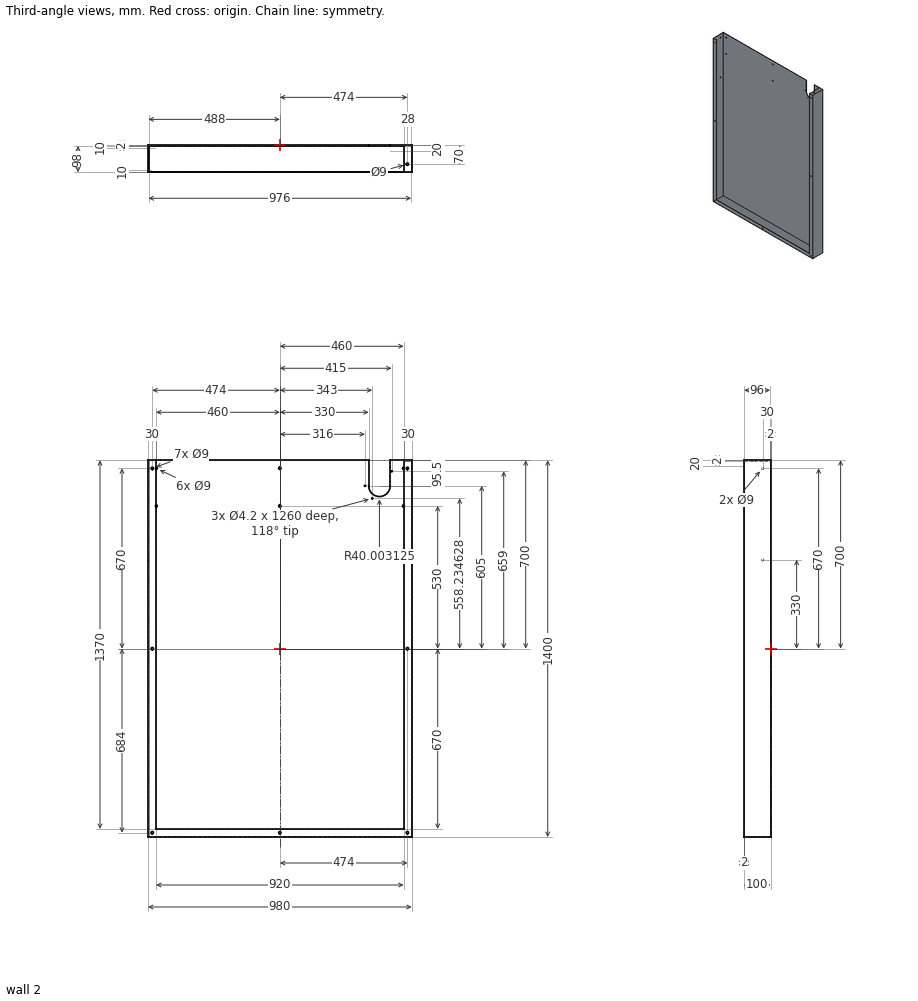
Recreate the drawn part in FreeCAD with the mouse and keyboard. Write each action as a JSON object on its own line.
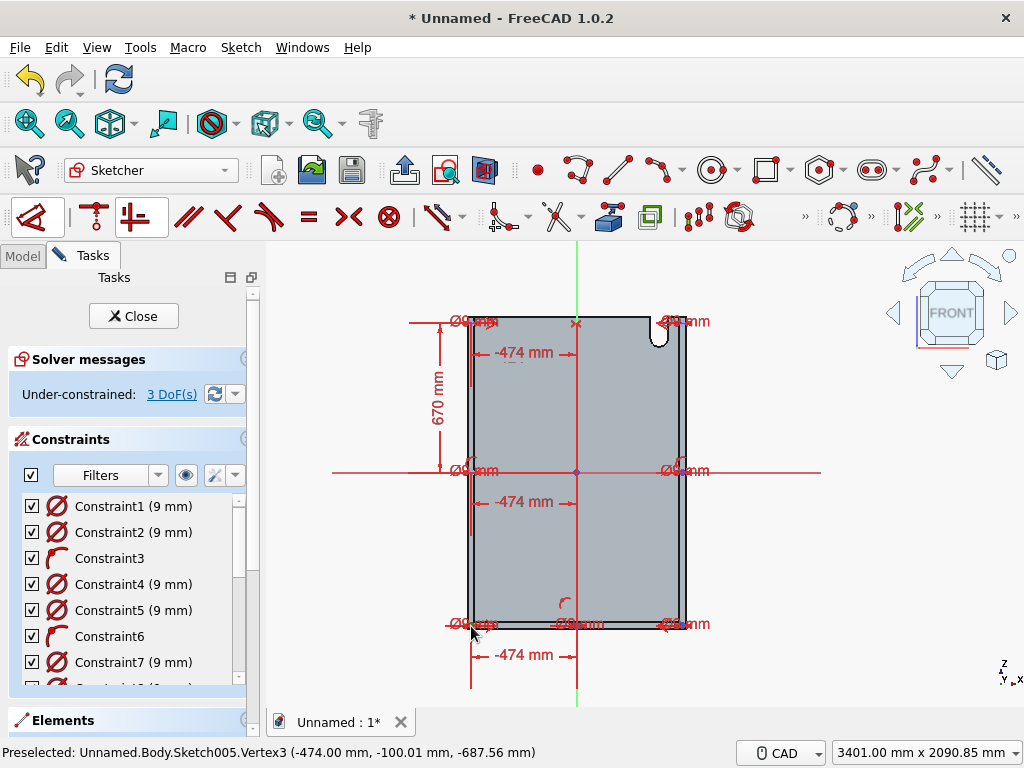
{"action": "key", "text": "i"}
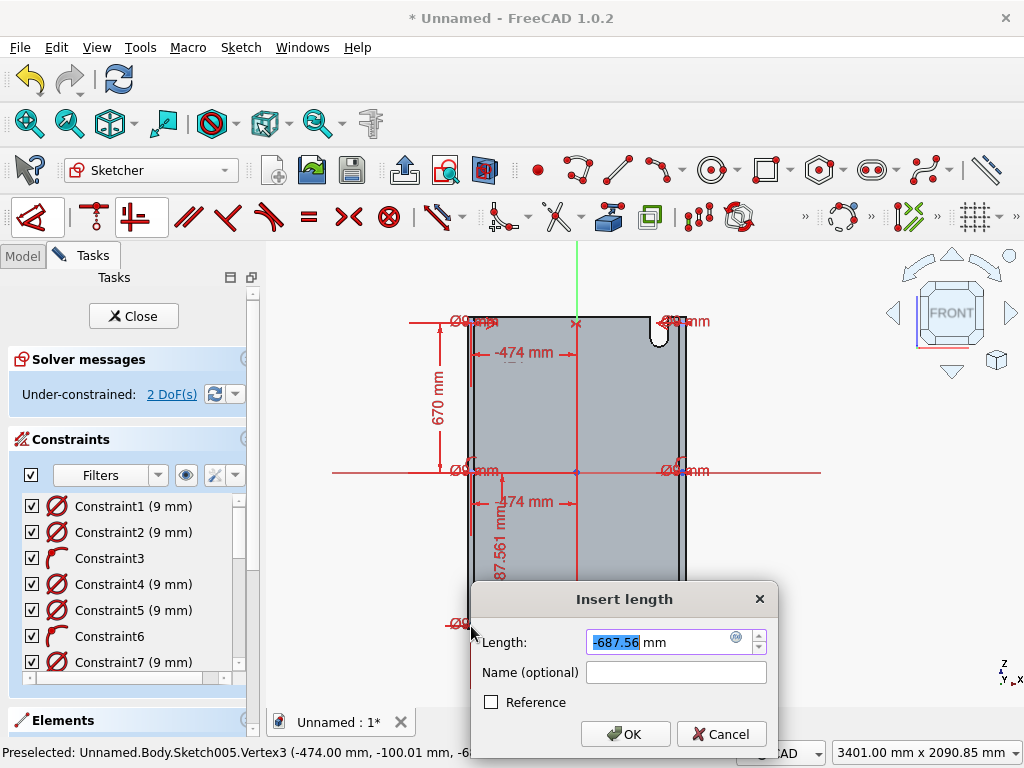
{"action": "type", "text": "-684"}
{"action": "key", "text": "Return"}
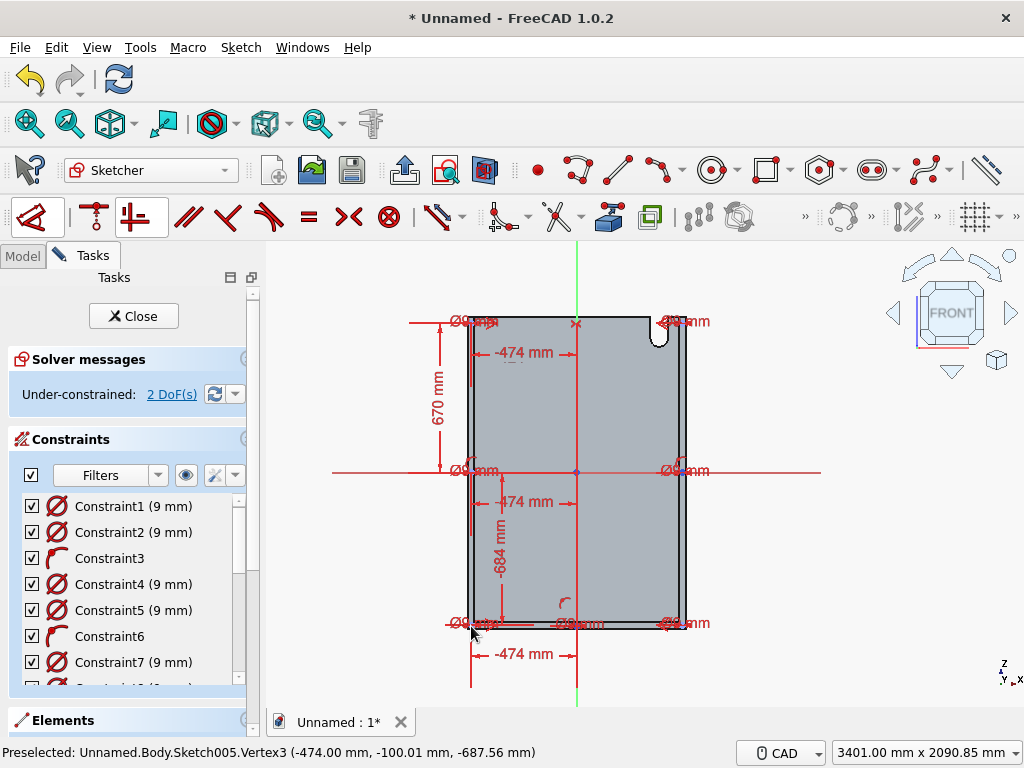
{"action": "left_click", "coordinate": [577, 626]}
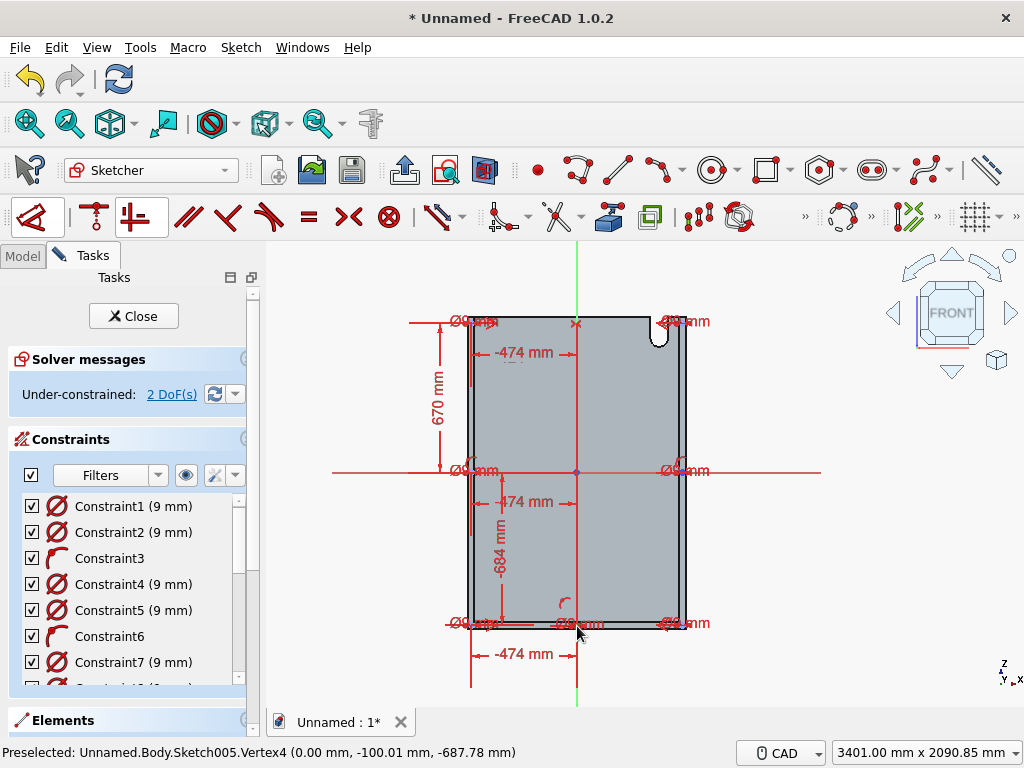
{"action": "key", "text": "i"}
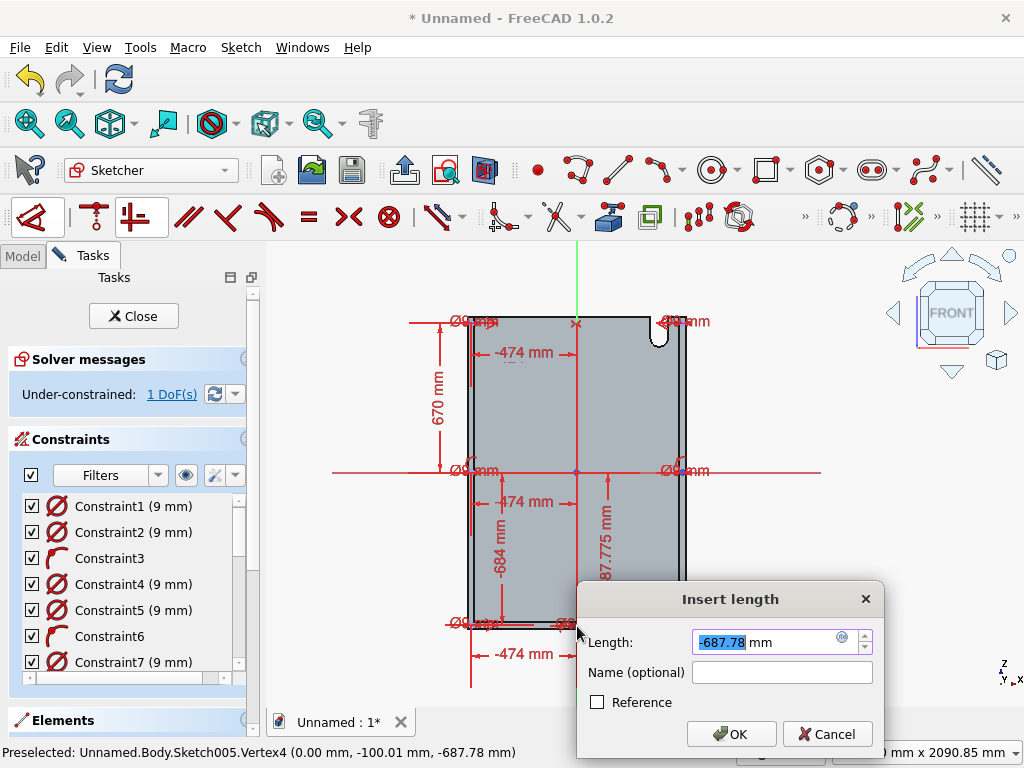
{"action": "type", "text": "-684"}
{"action": "key", "text": "Return"}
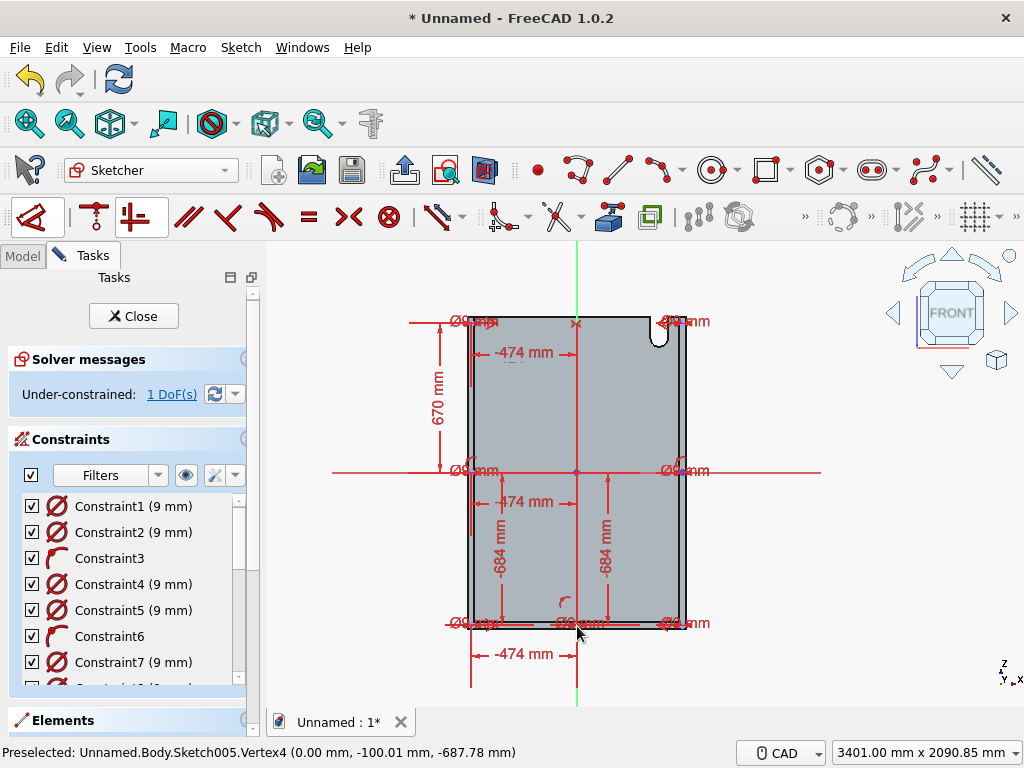
{"action": "left_click", "coordinate": [682, 473]}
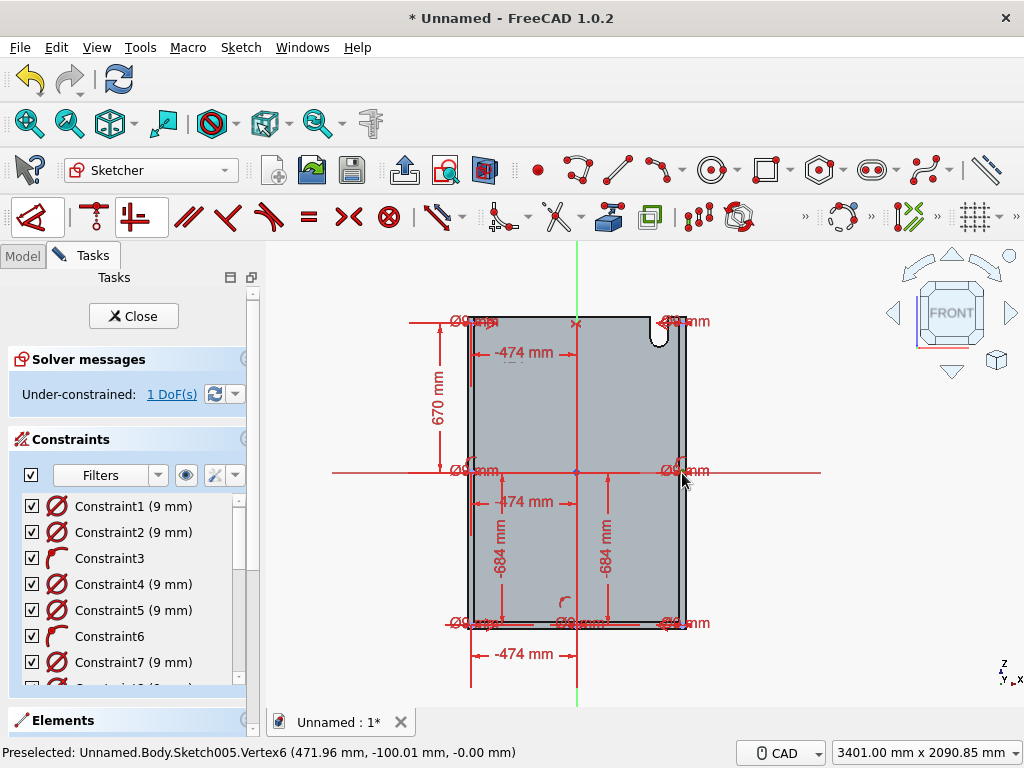
{"action": "left_click", "coordinate": [58, 218]}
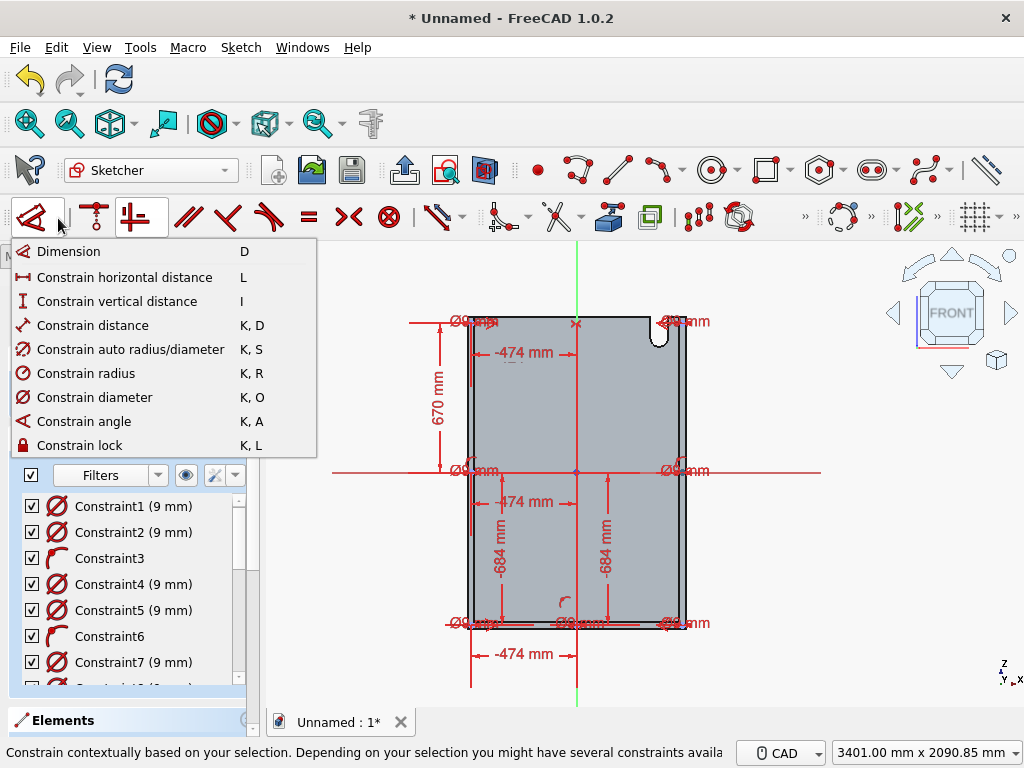
{"action": "left_click", "coordinate": [164, 277]}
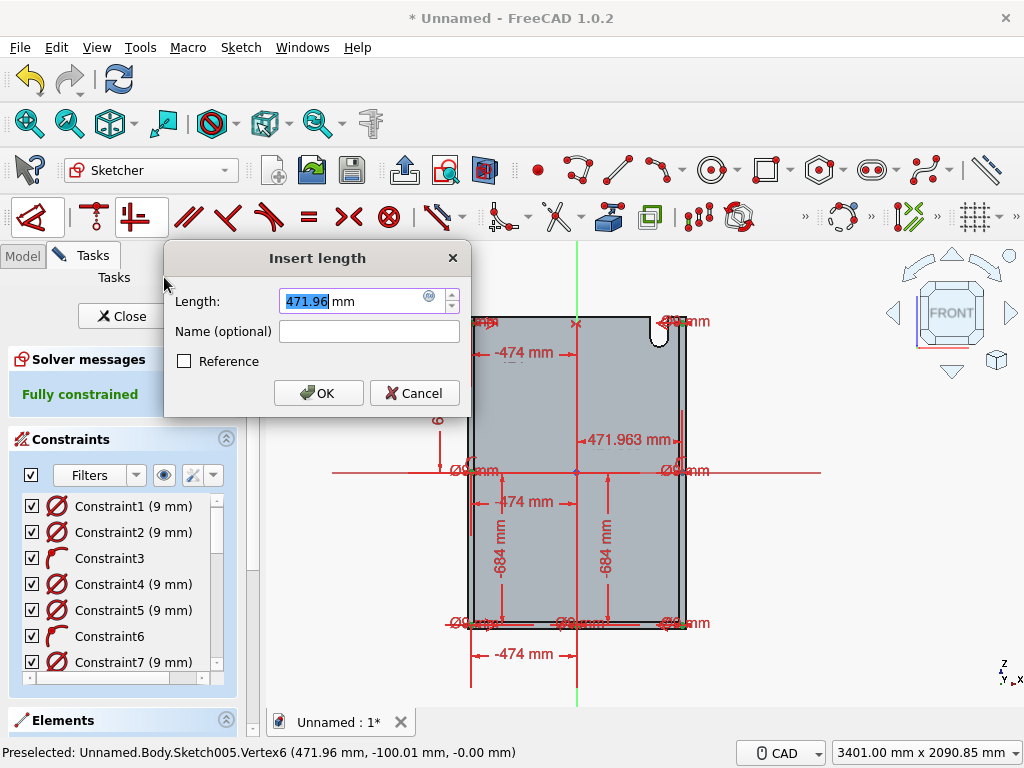
{"action": "type", "text": "474"}
{"action": "key", "text": "Return"}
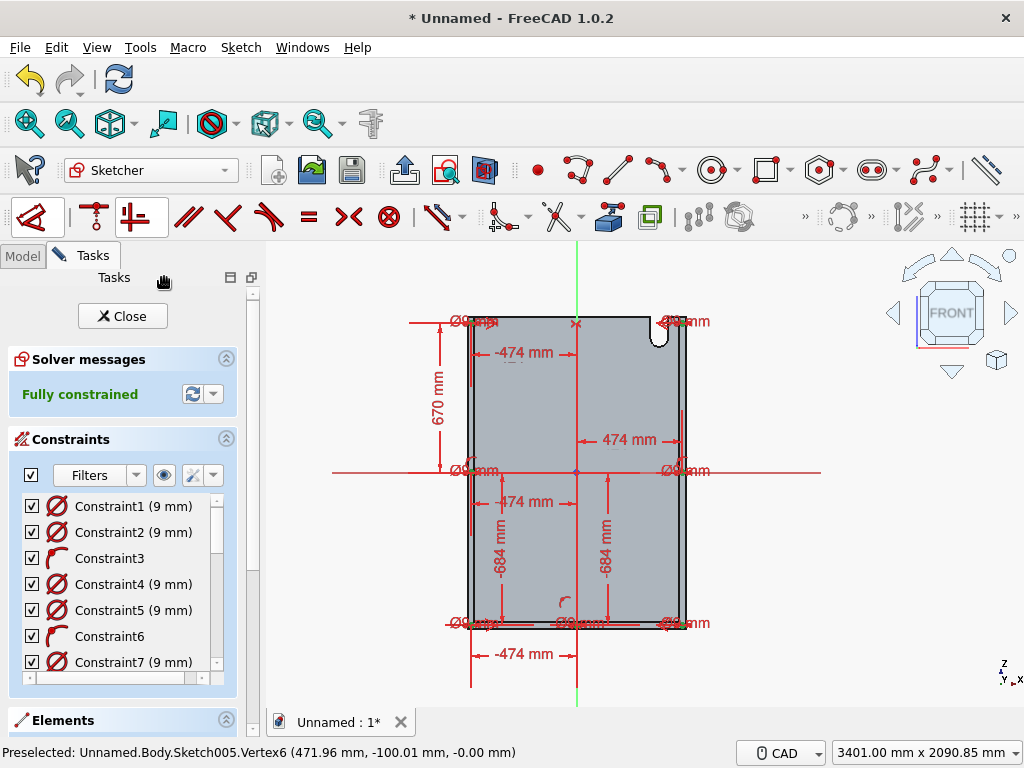
{"action": "left_click", "coordinate": [123, 316]}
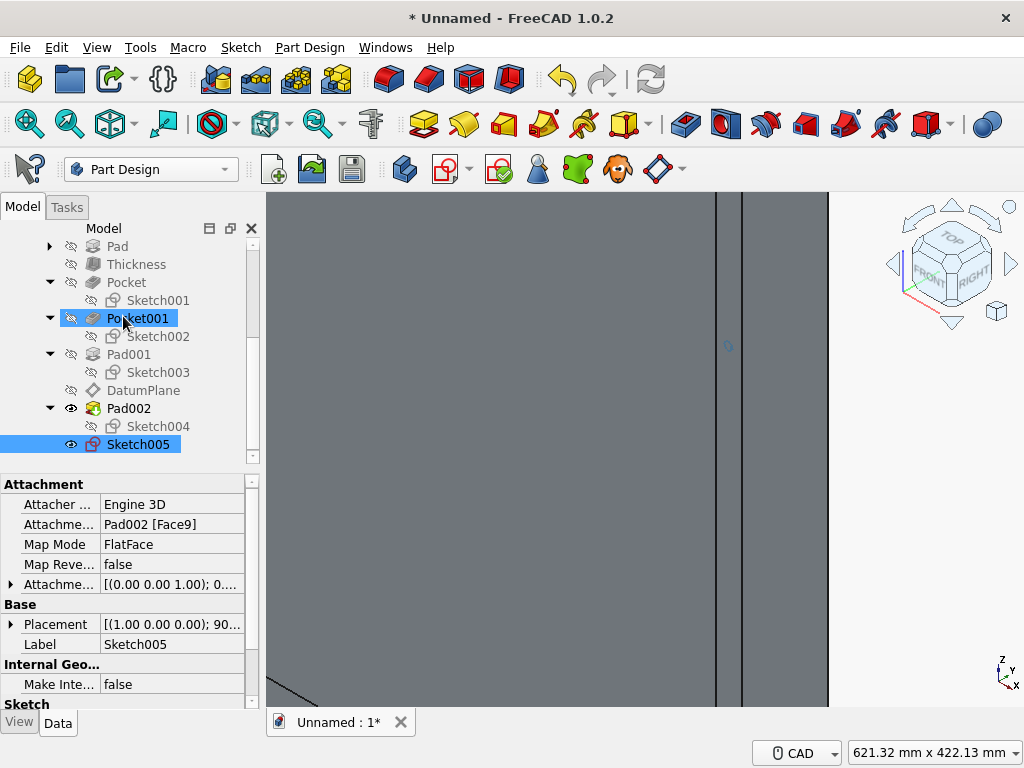
{"action": "left_click", "coordinate": [686, 124]}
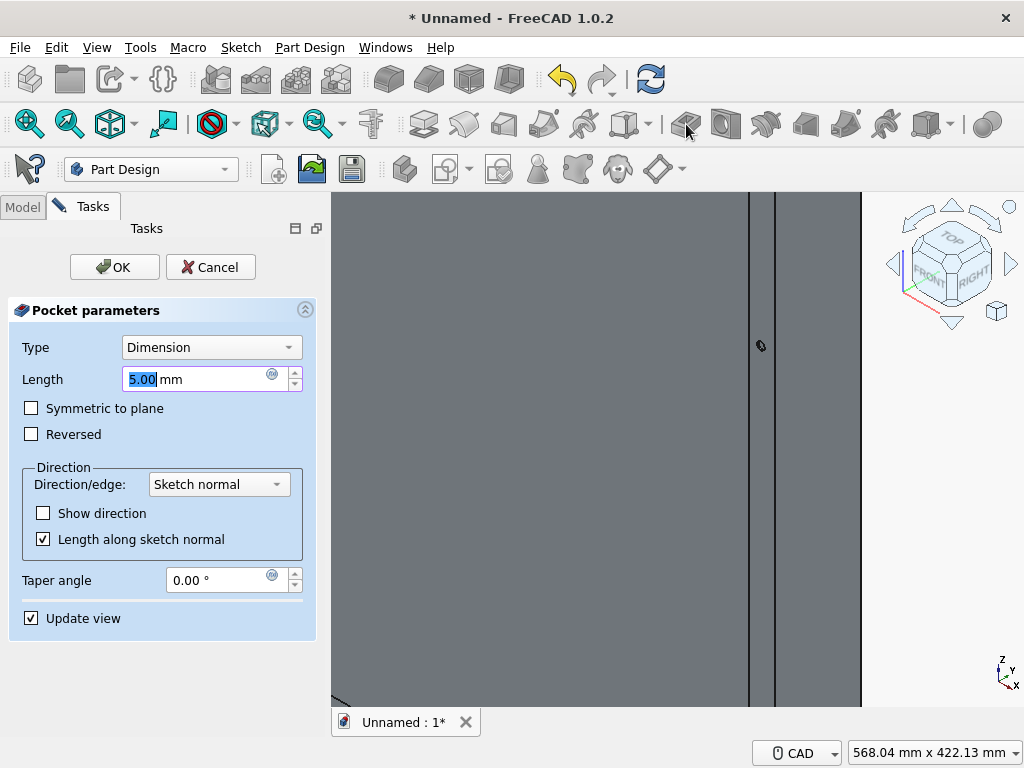
{"action": "type", "text": "10"}
{"action": "key", "text": "Tab"}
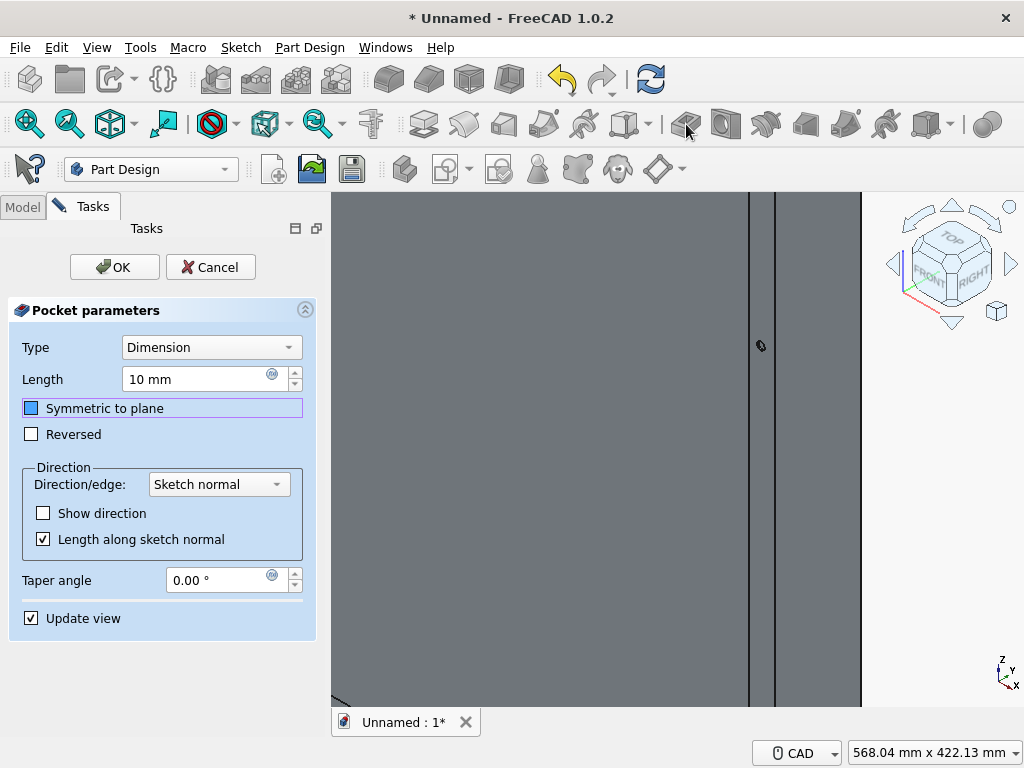
{"action": "left_click", "coordinate": [115, 267]}